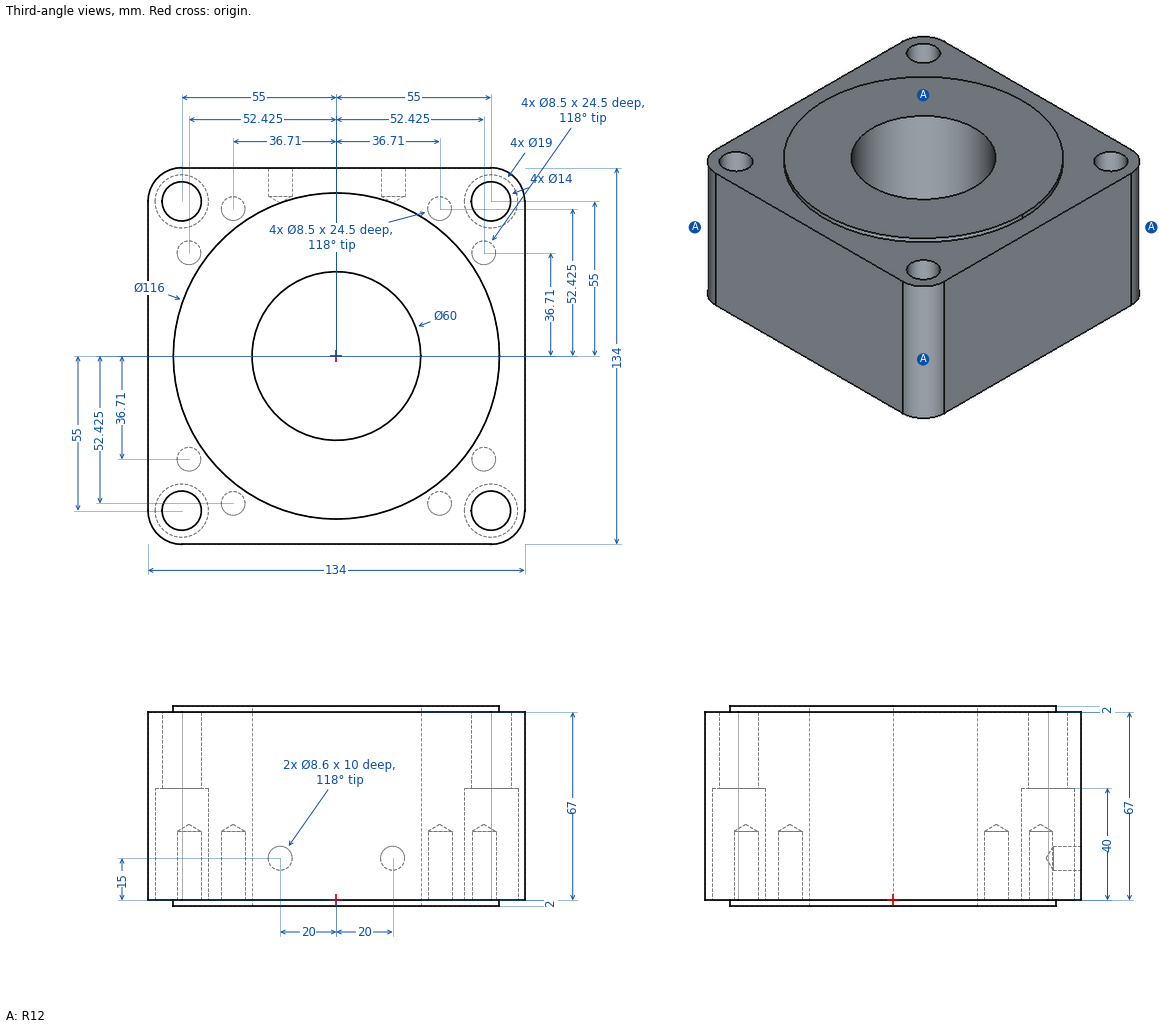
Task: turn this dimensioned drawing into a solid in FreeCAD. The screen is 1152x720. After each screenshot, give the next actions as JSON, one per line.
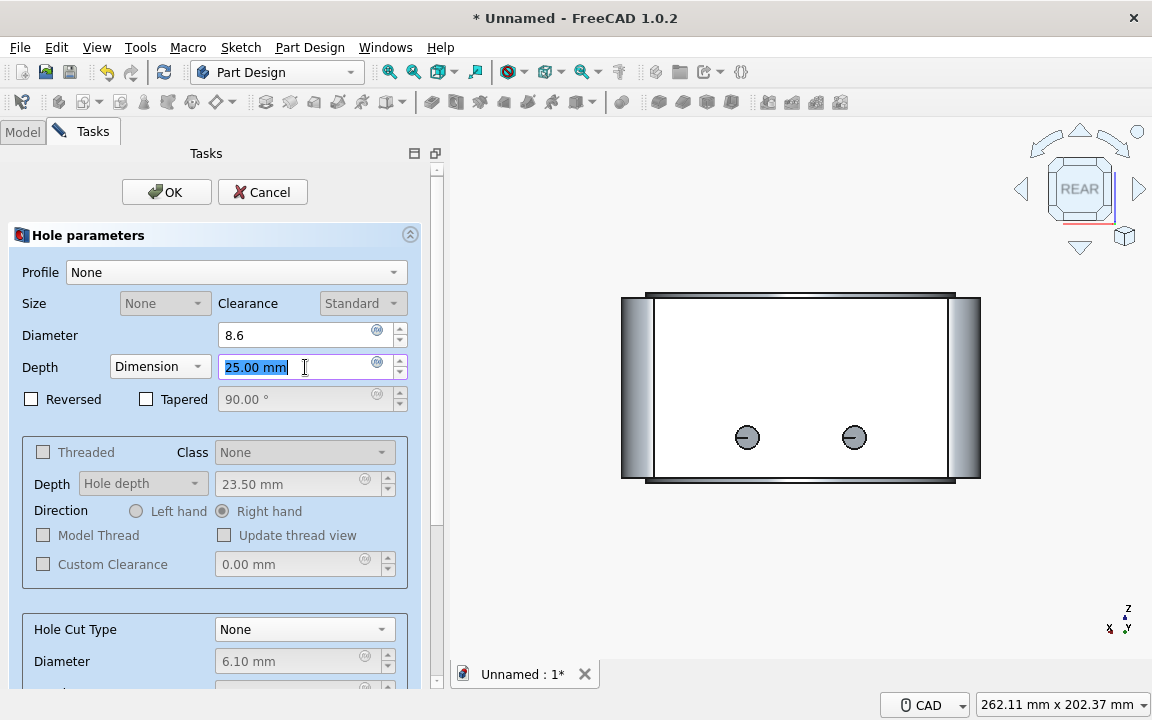
{"action": "type", "text": "10"}
{"action": "key", "text": "Tab"}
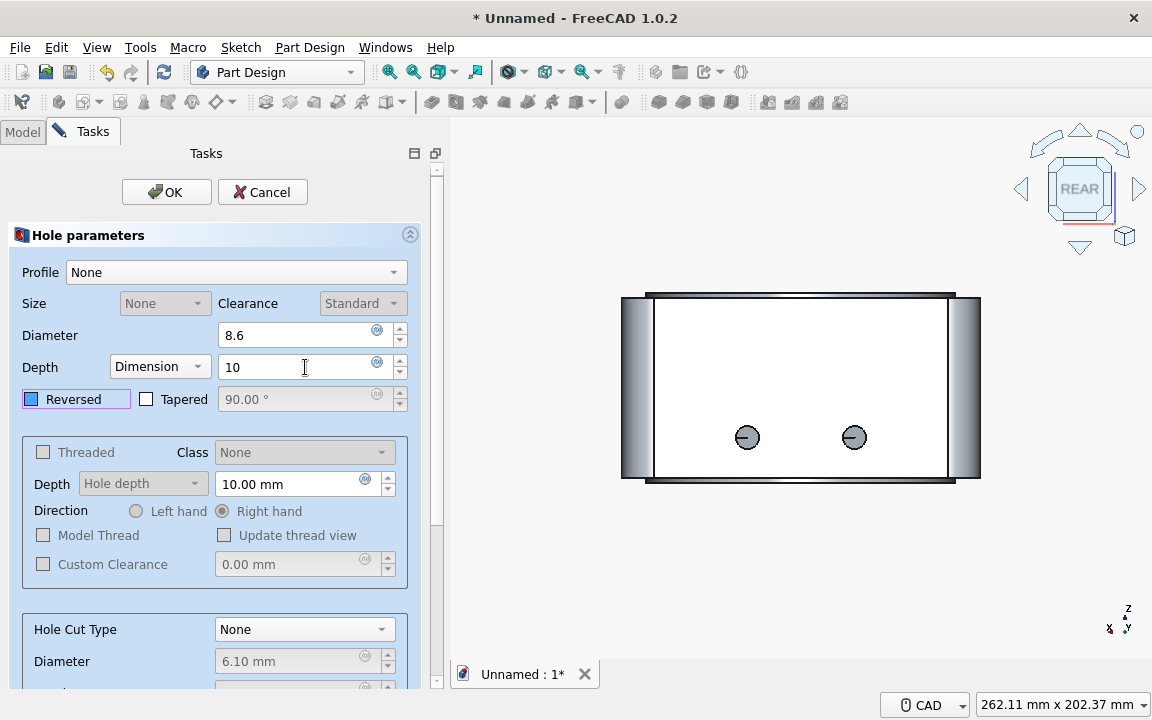
{"action": "left_click", "coordinate": [167, 192]}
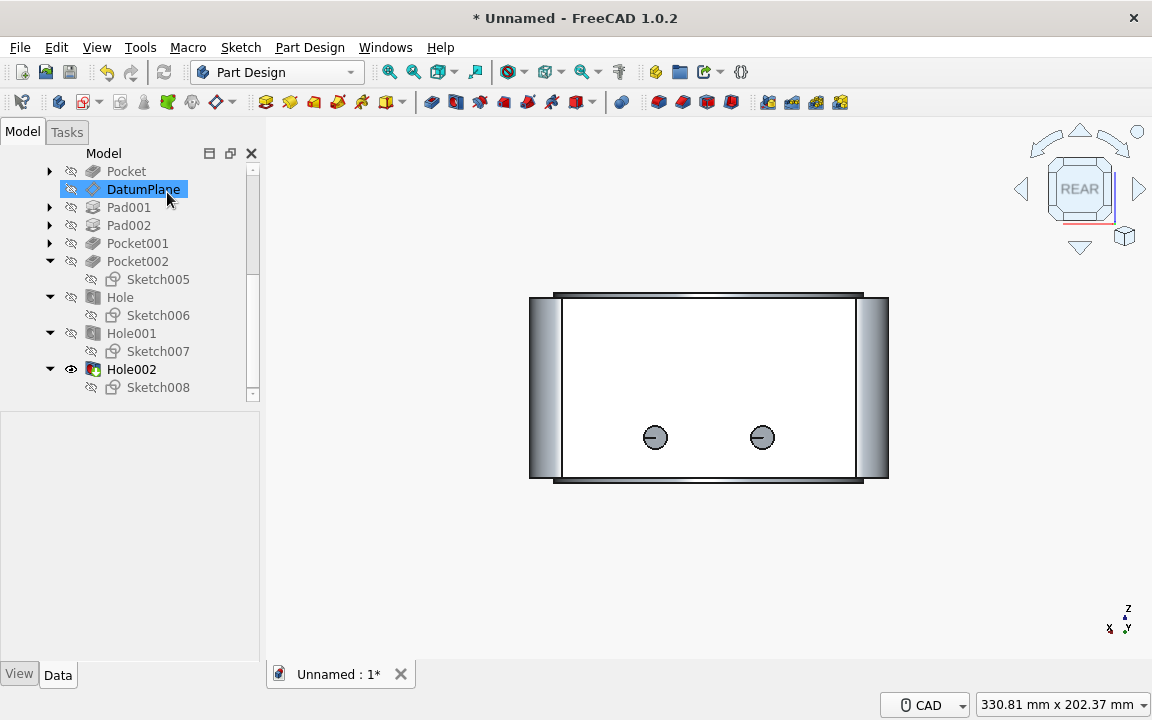
{"action": "key", "text": "0"}